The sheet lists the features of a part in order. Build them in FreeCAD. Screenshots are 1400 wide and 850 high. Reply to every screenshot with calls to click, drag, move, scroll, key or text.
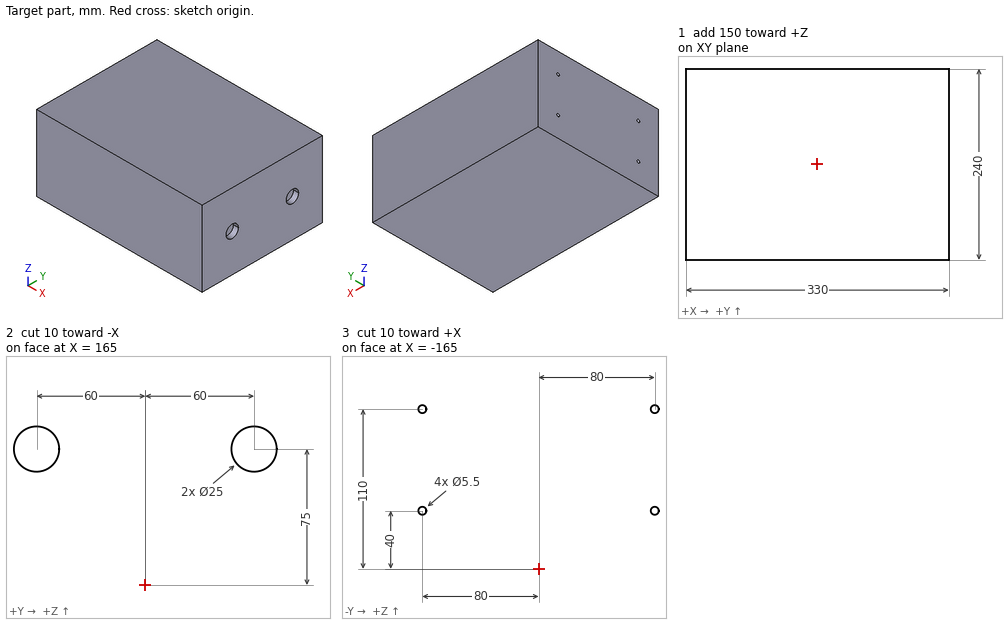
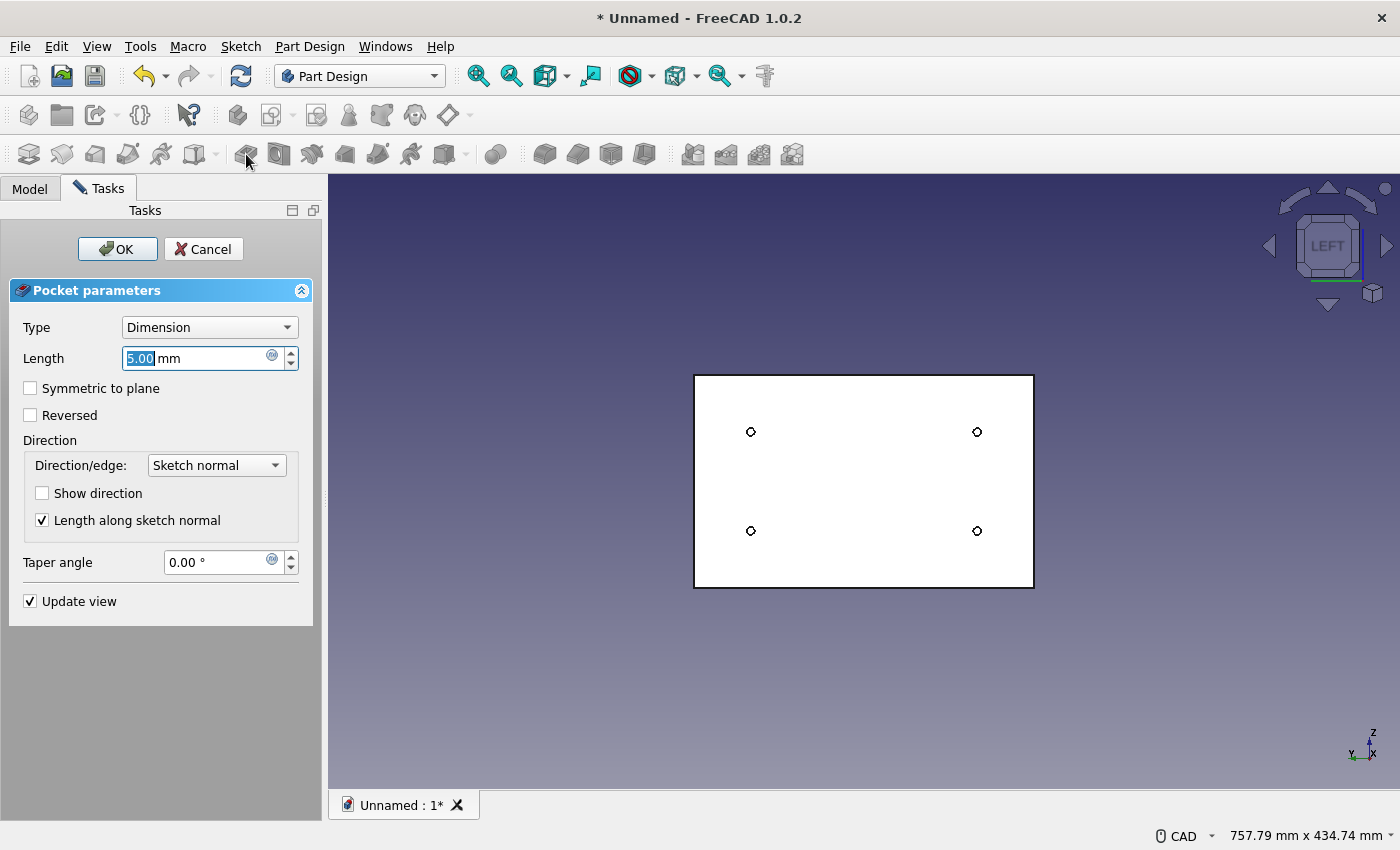
text(10)
key(Tab)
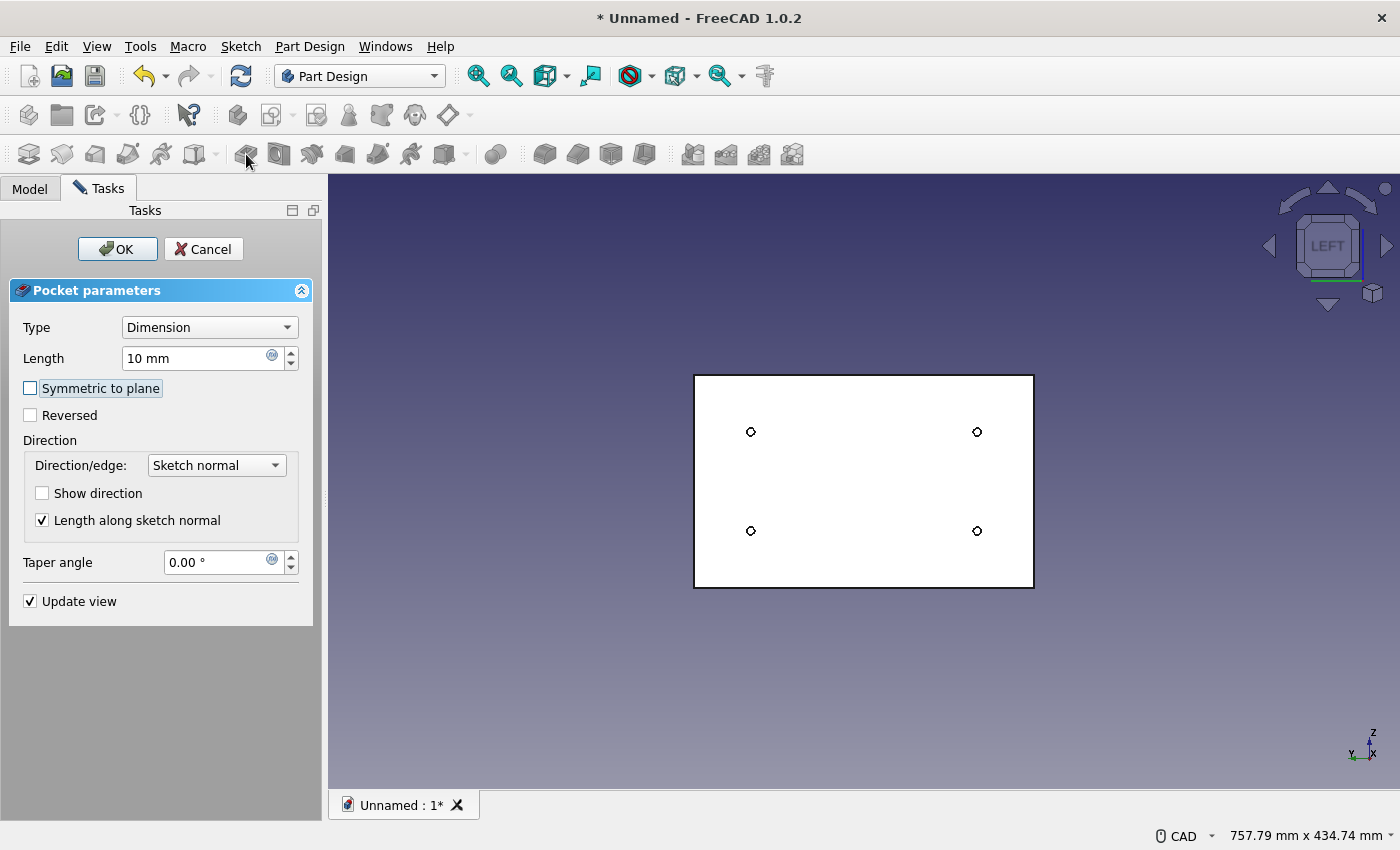
click(118, 249)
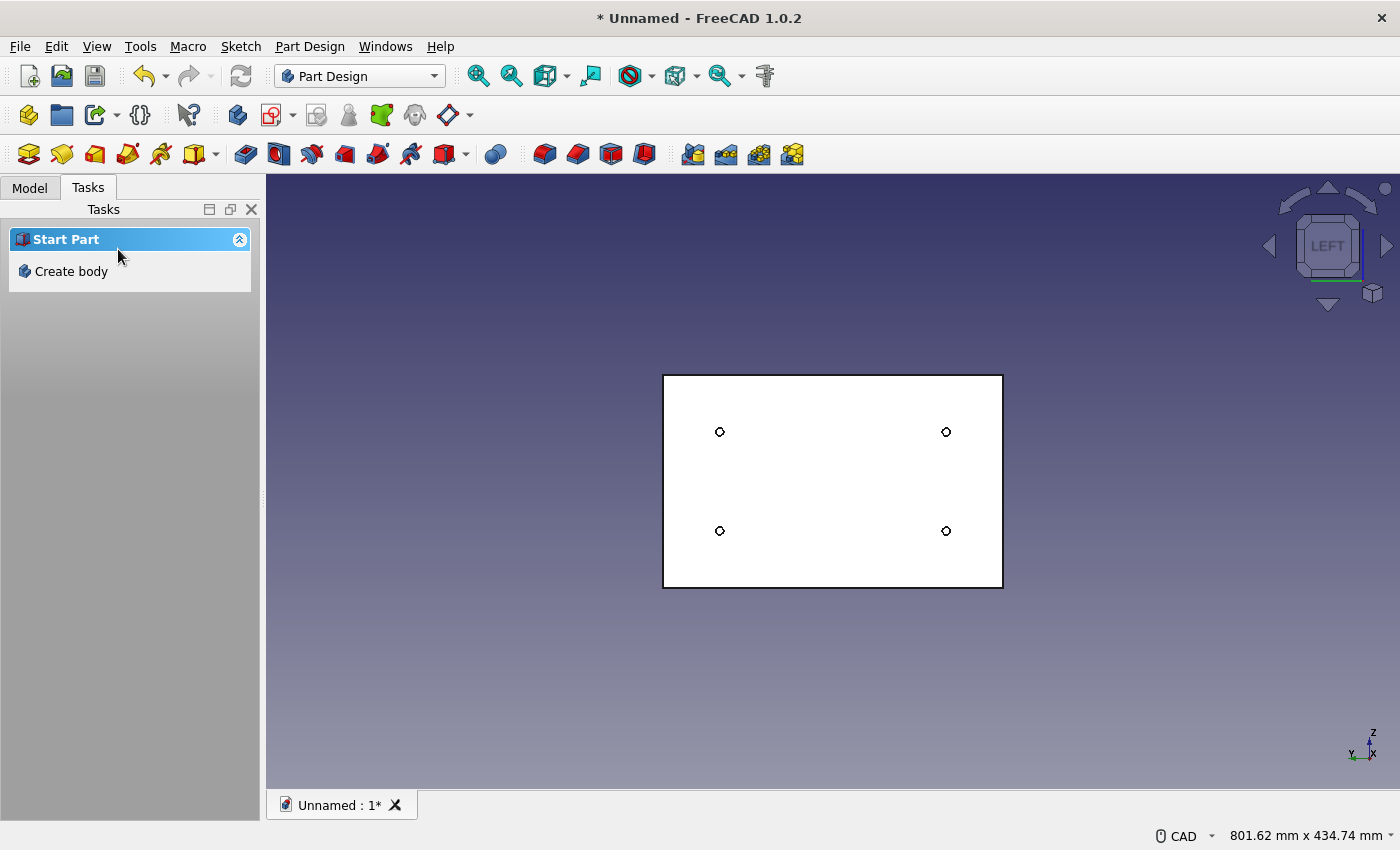
key(0)